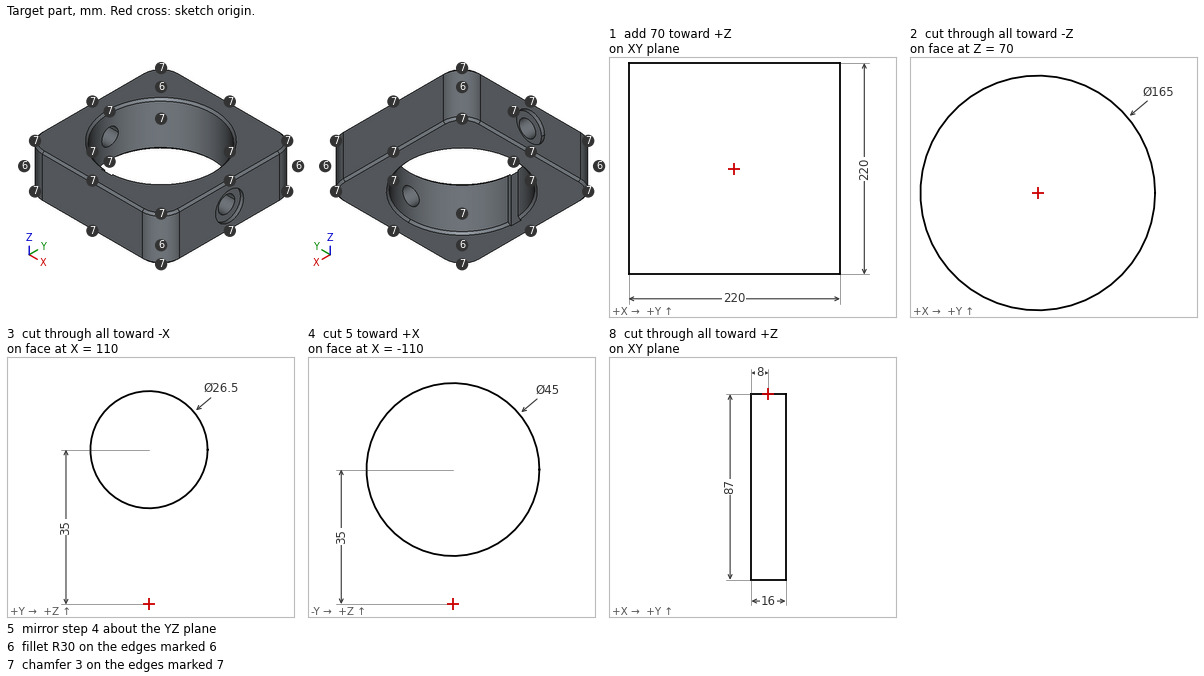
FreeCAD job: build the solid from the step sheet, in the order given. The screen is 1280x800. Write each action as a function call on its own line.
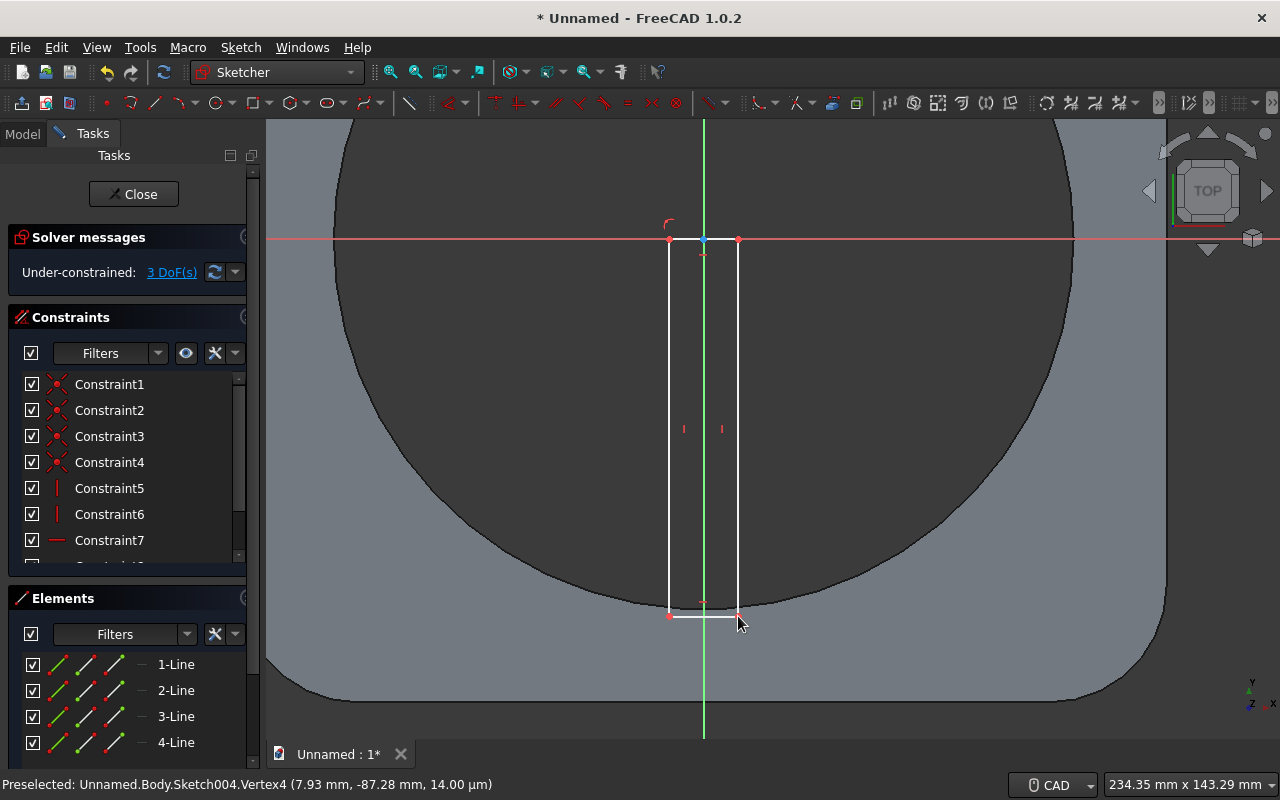
key(d)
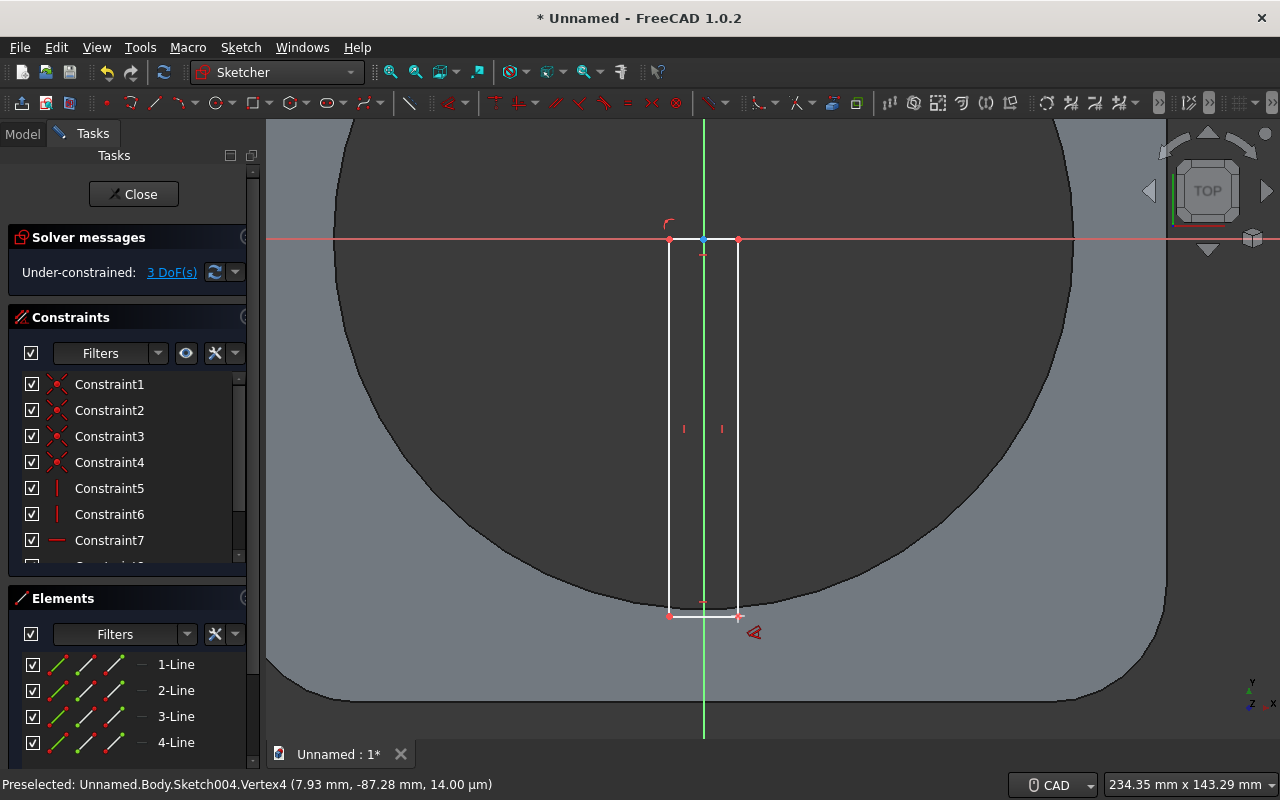
click(669, 353)
click(635, 428)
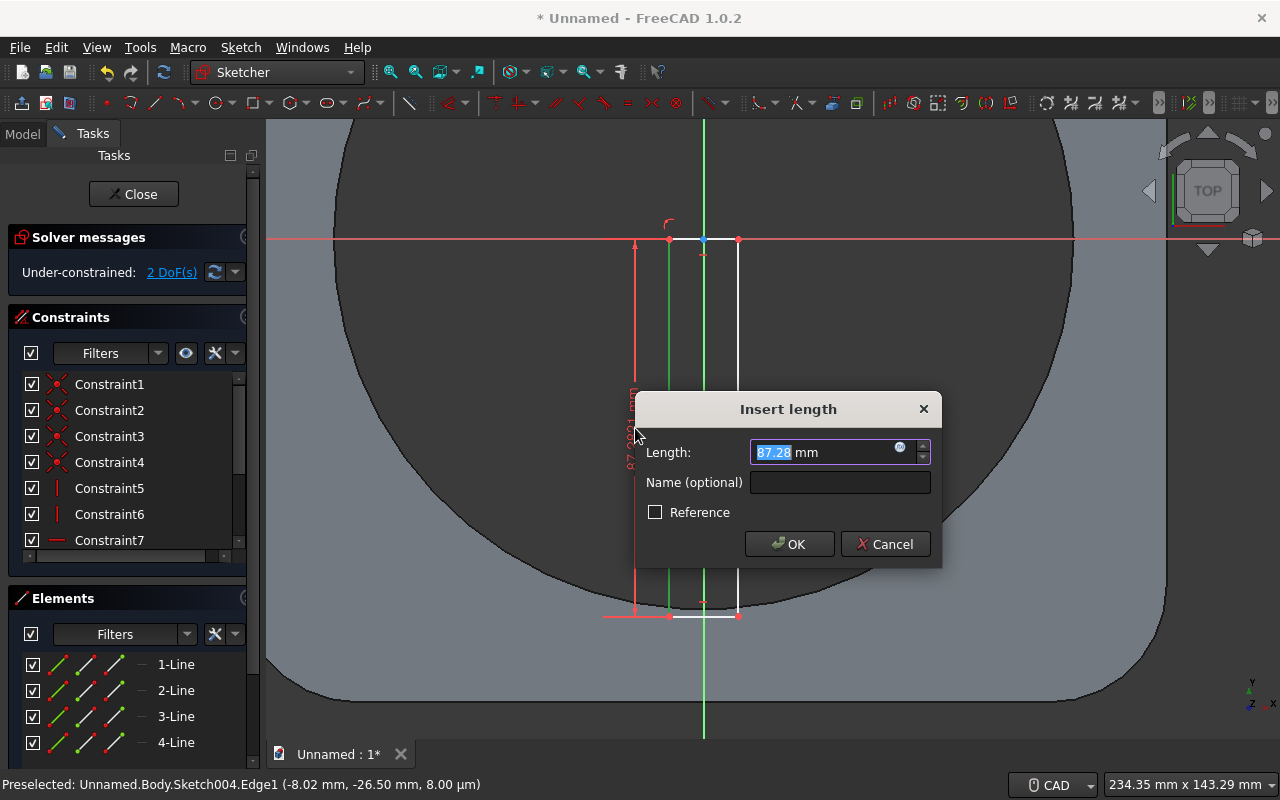
text(87)
key(Return)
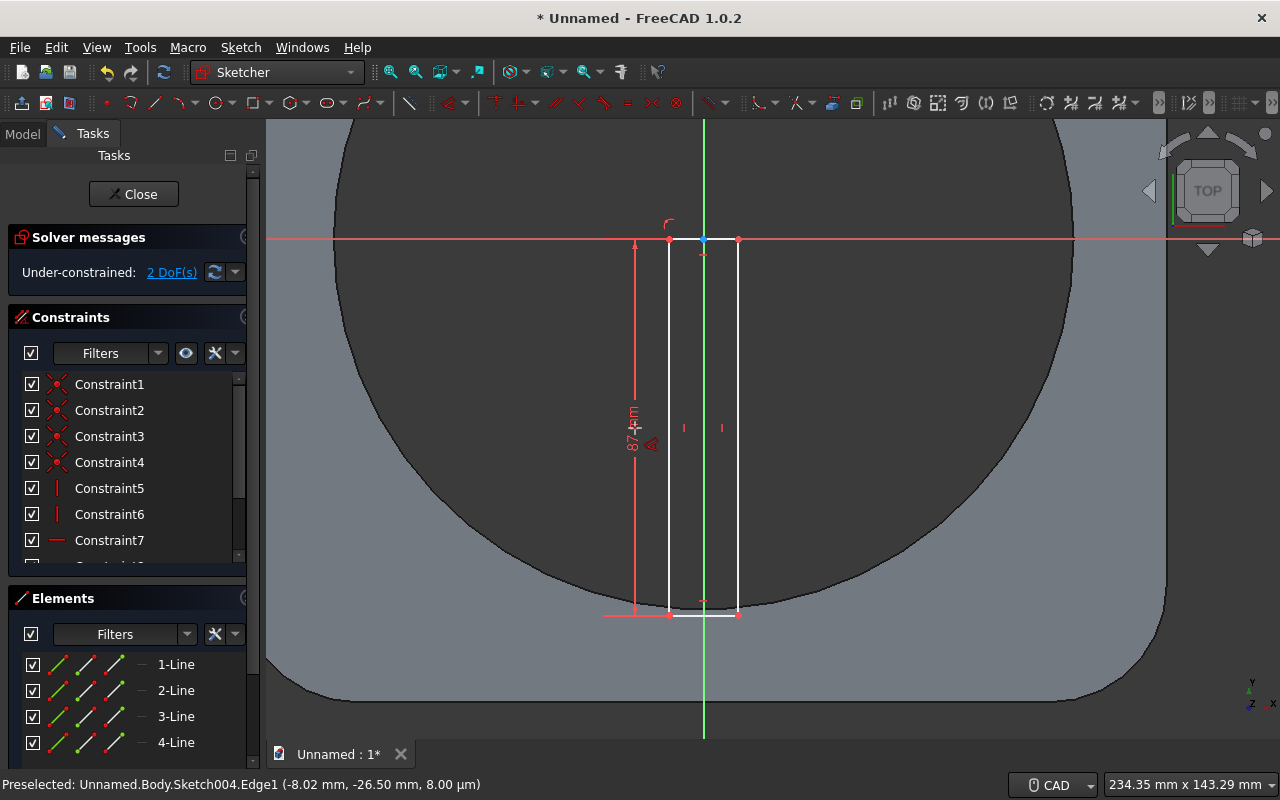
click(690, 616)
click(688, 650)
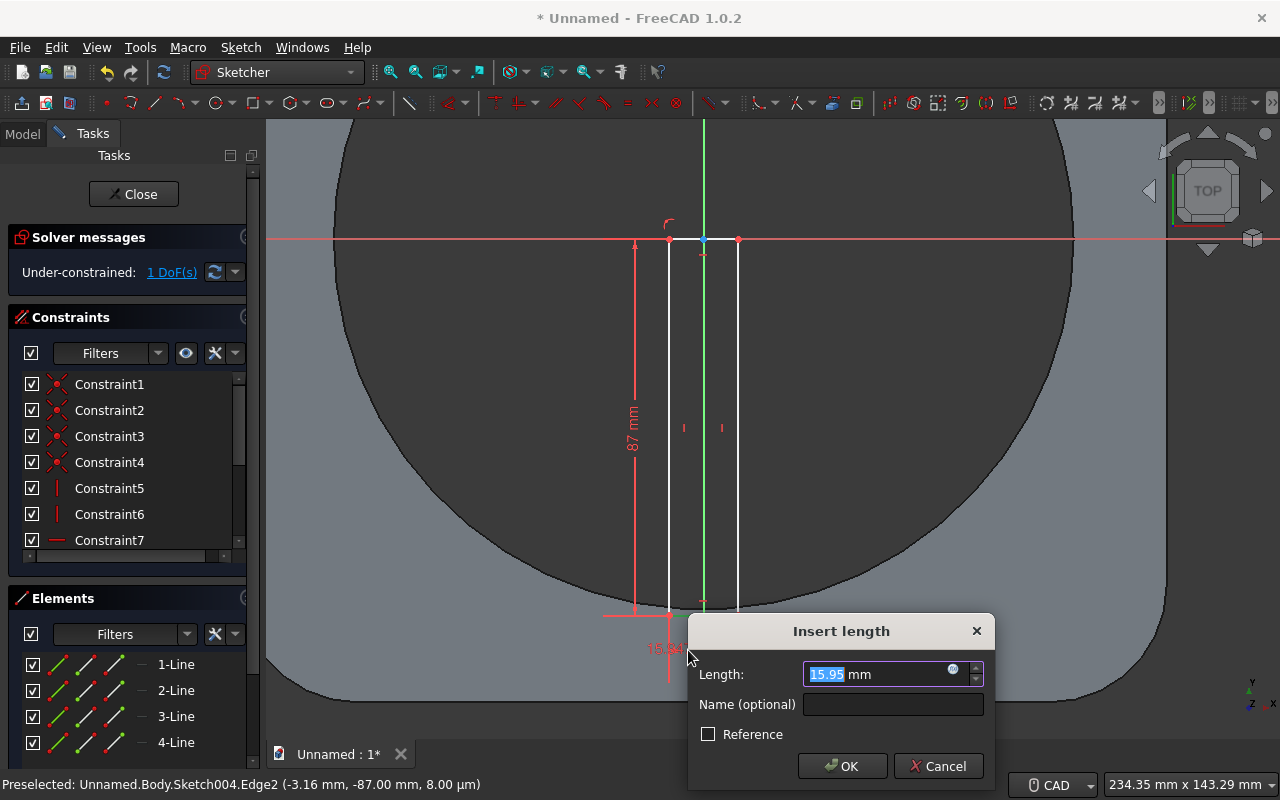
text(16)
key(Return)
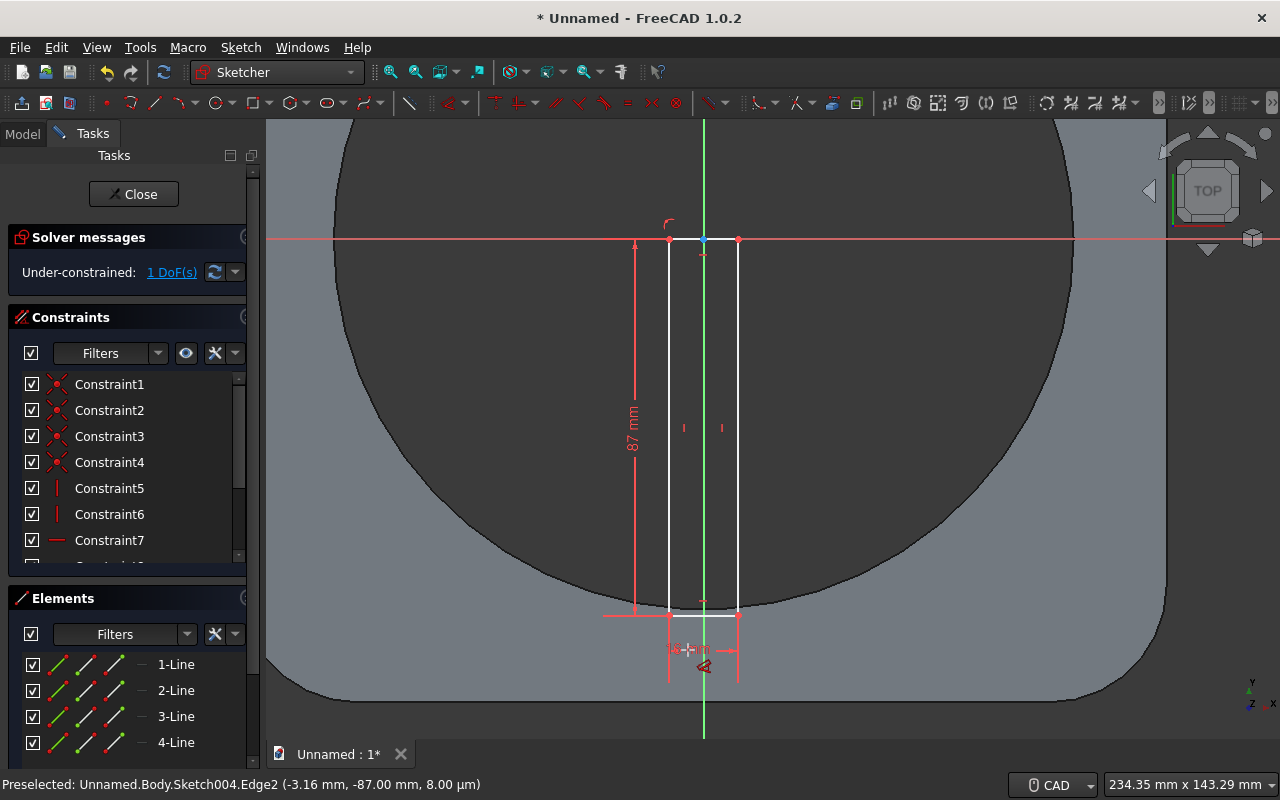
click(669, 239)
click(686, 205)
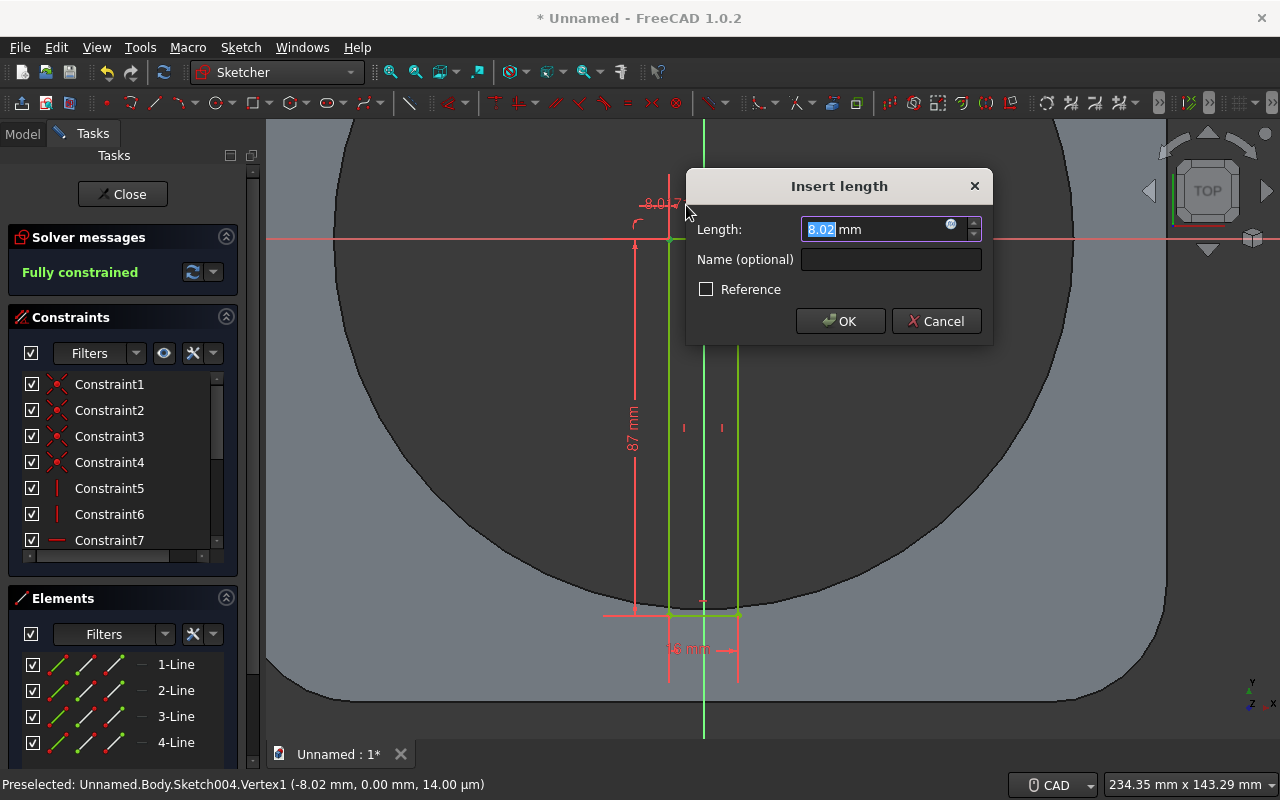
text(8)
key(Return)
key(Escape)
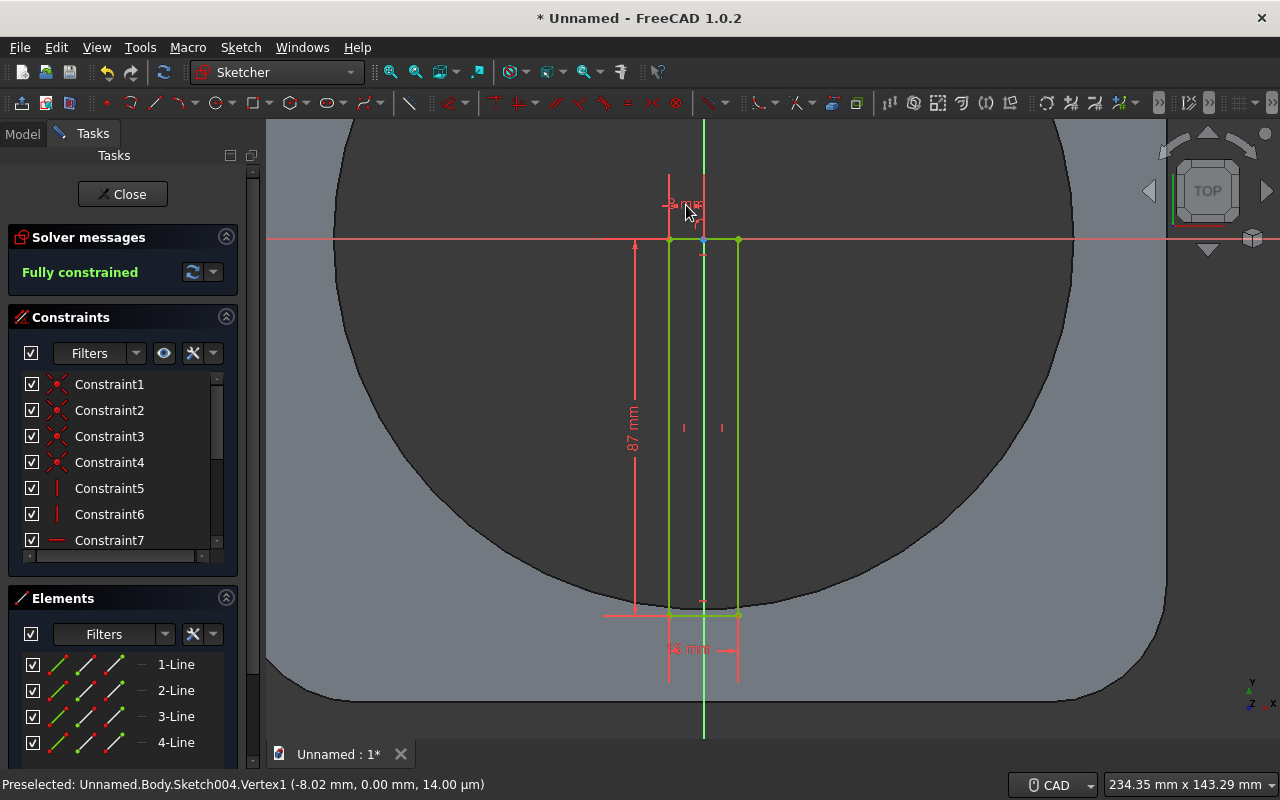
click(123, 194)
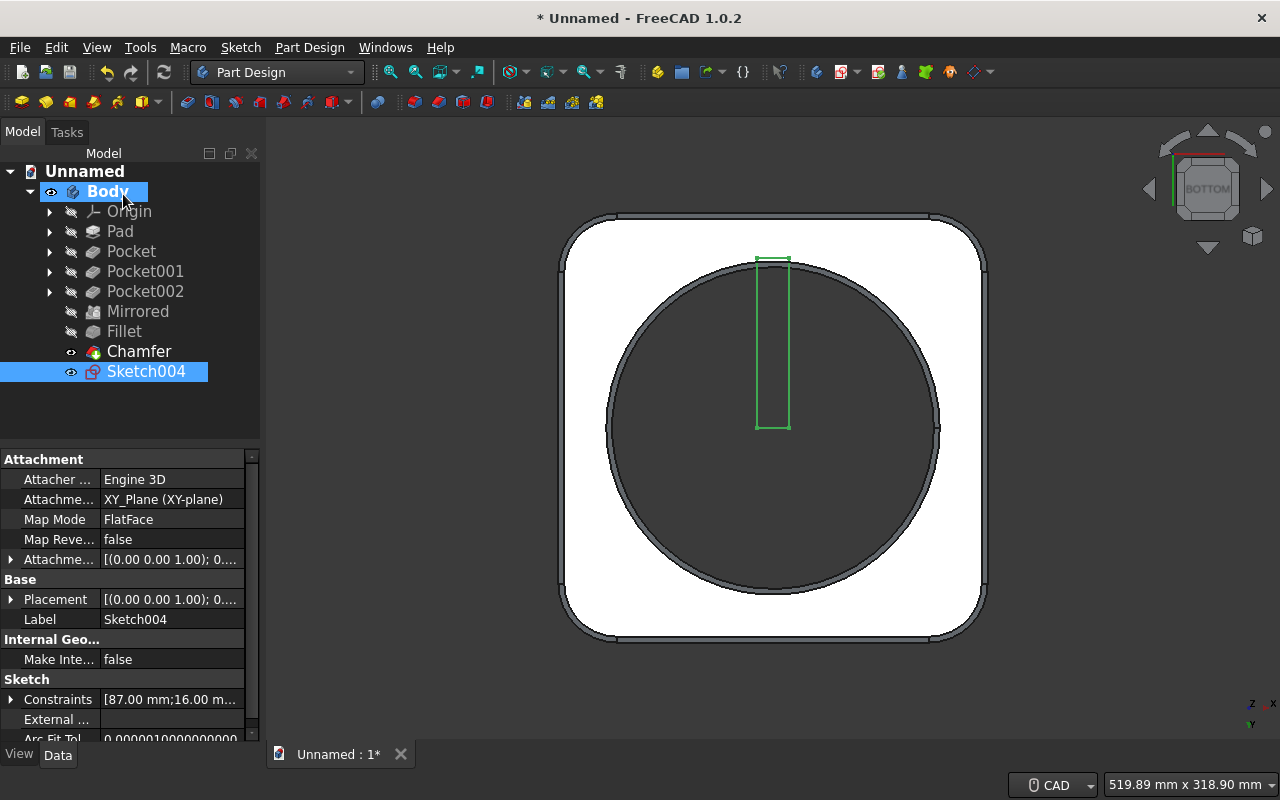
click(188, 102)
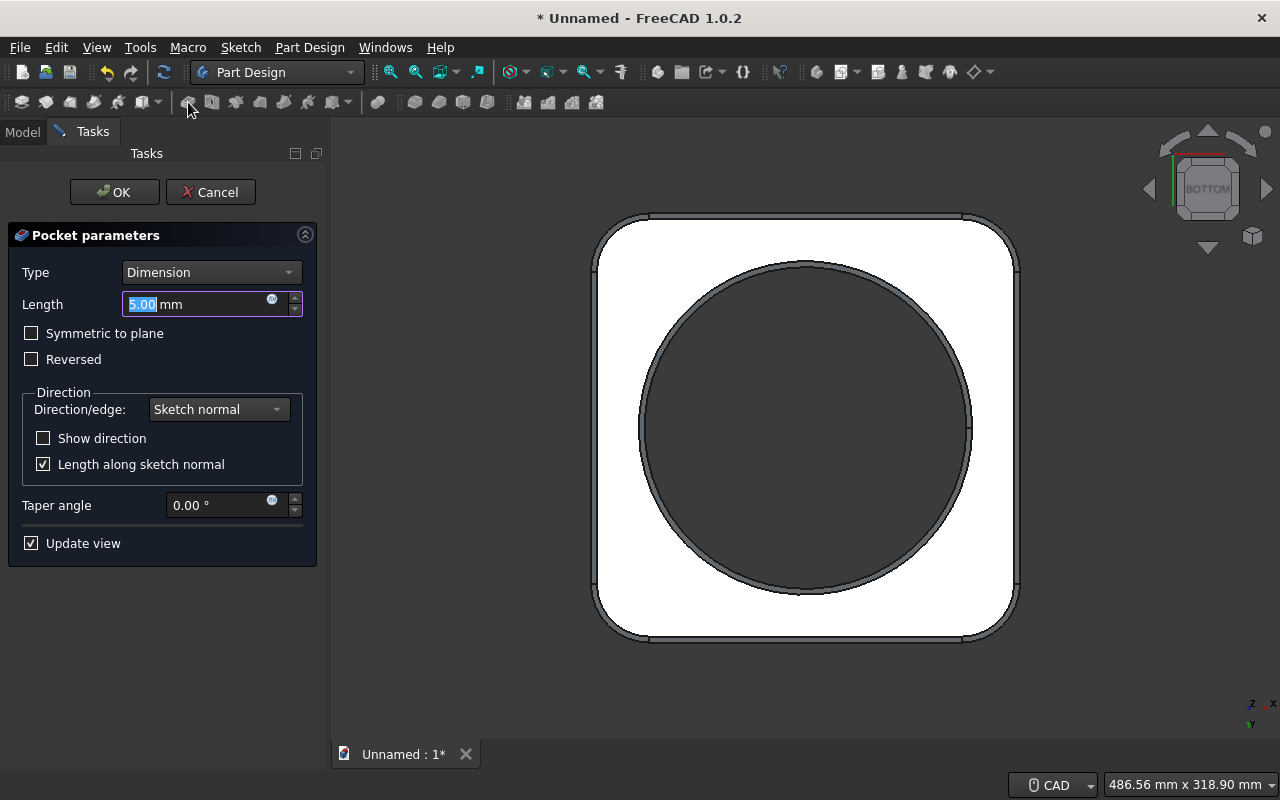
click(212, 272)